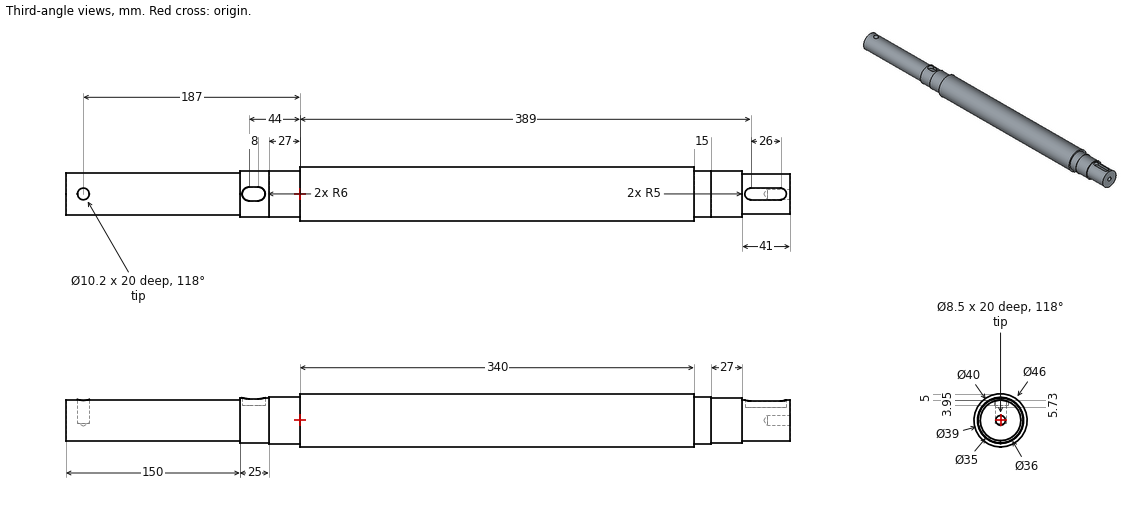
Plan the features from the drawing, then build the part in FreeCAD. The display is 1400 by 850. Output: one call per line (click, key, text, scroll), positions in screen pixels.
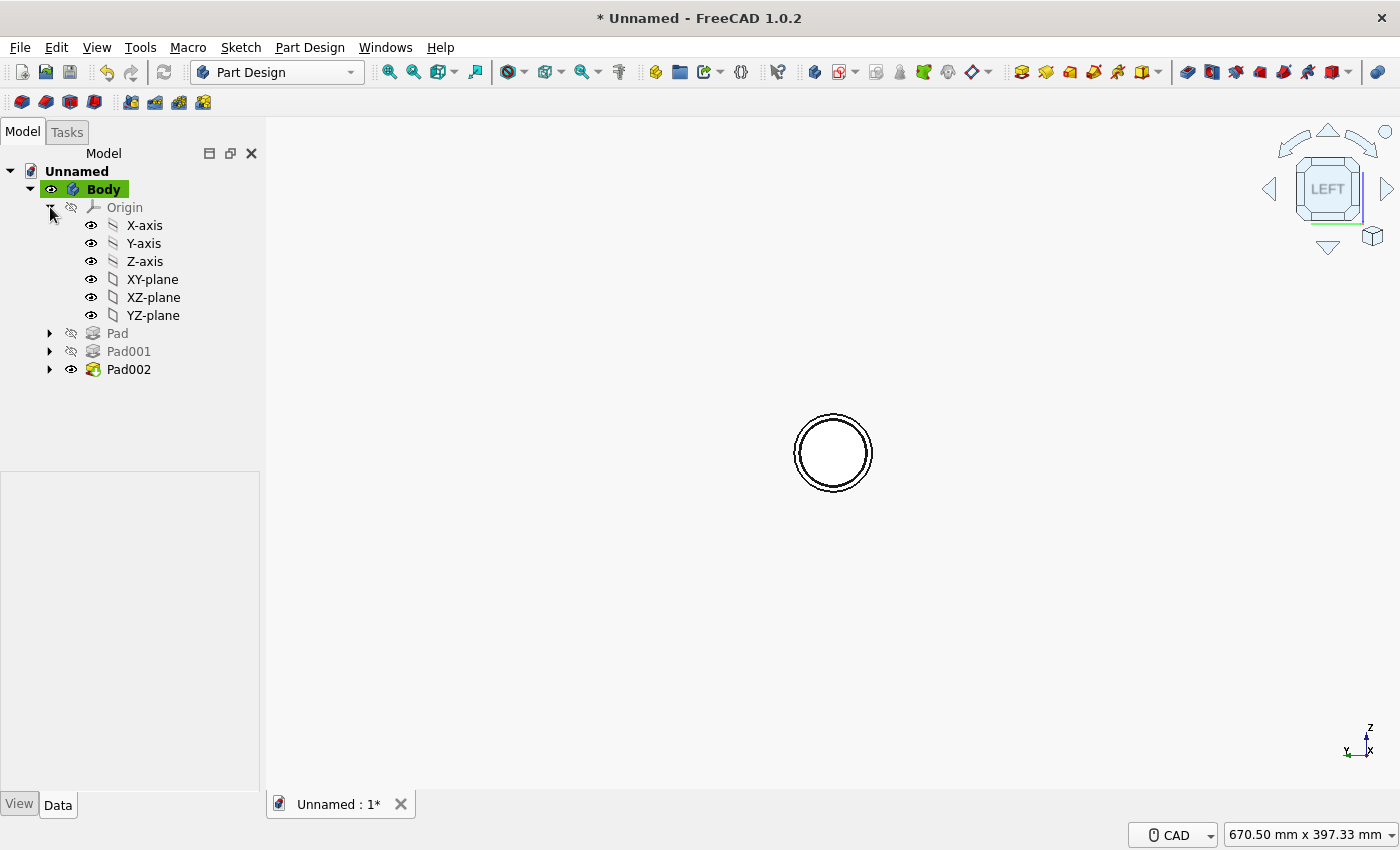
click(136, 315)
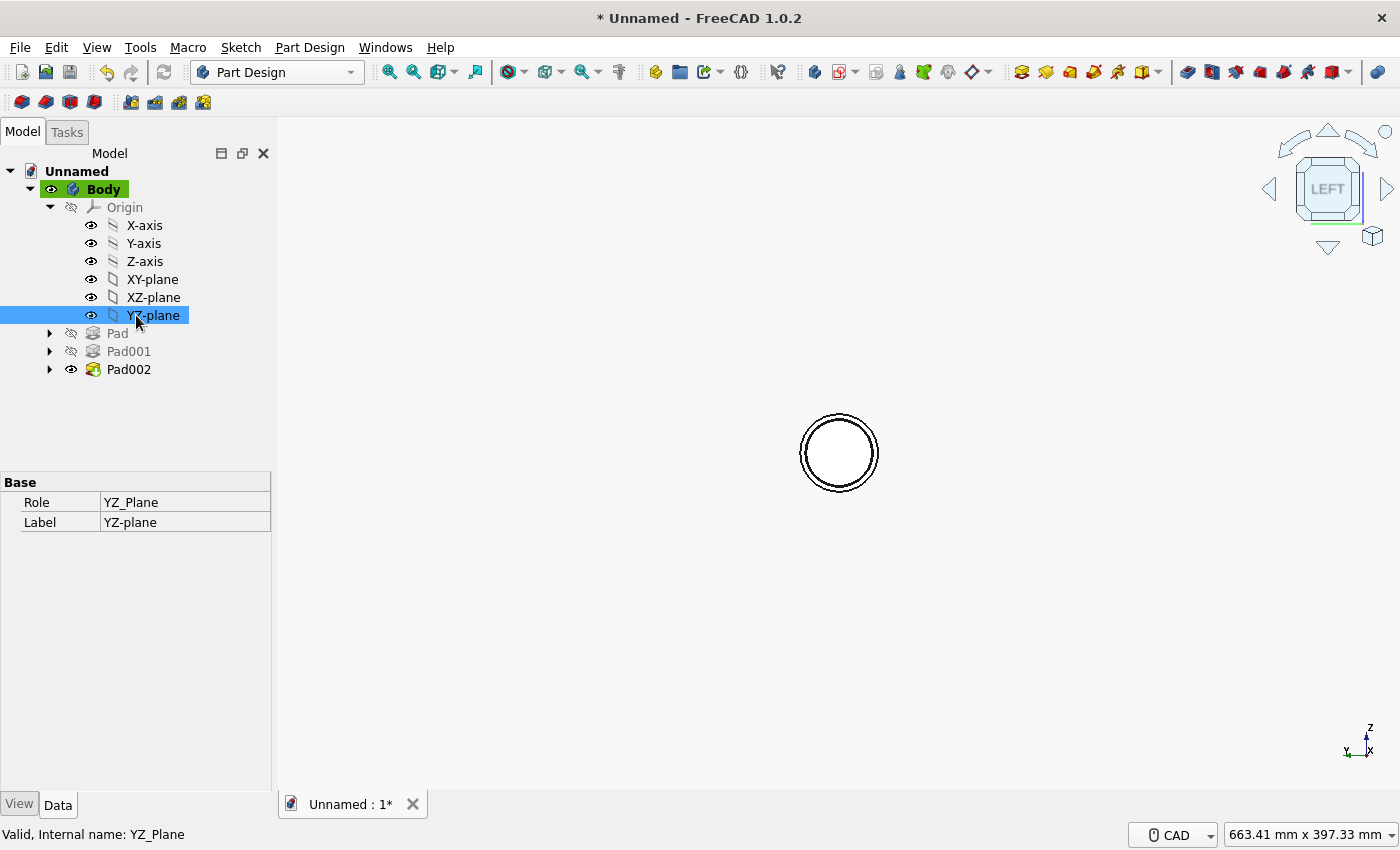
click(972, 72)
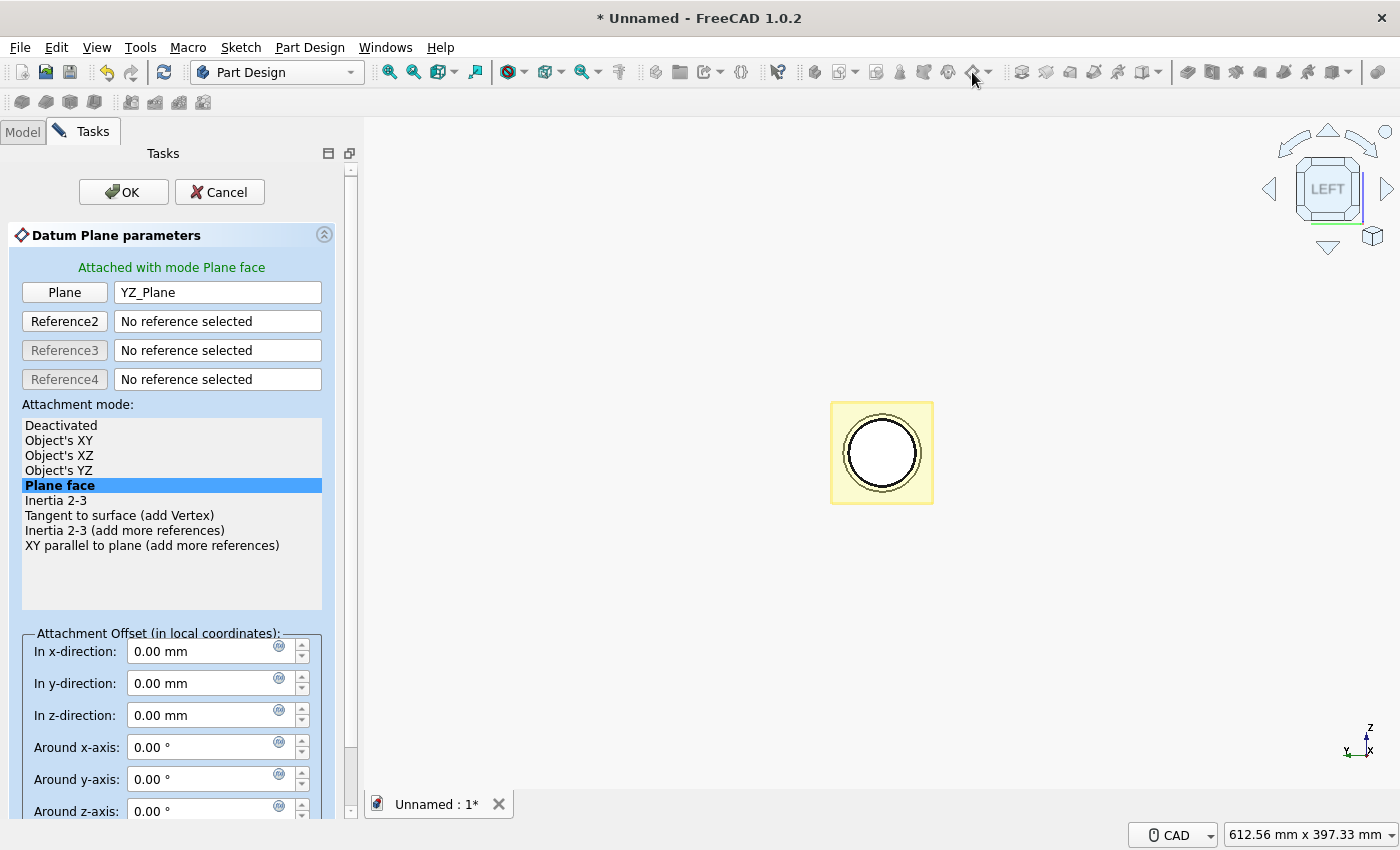
triple_click(210, 715)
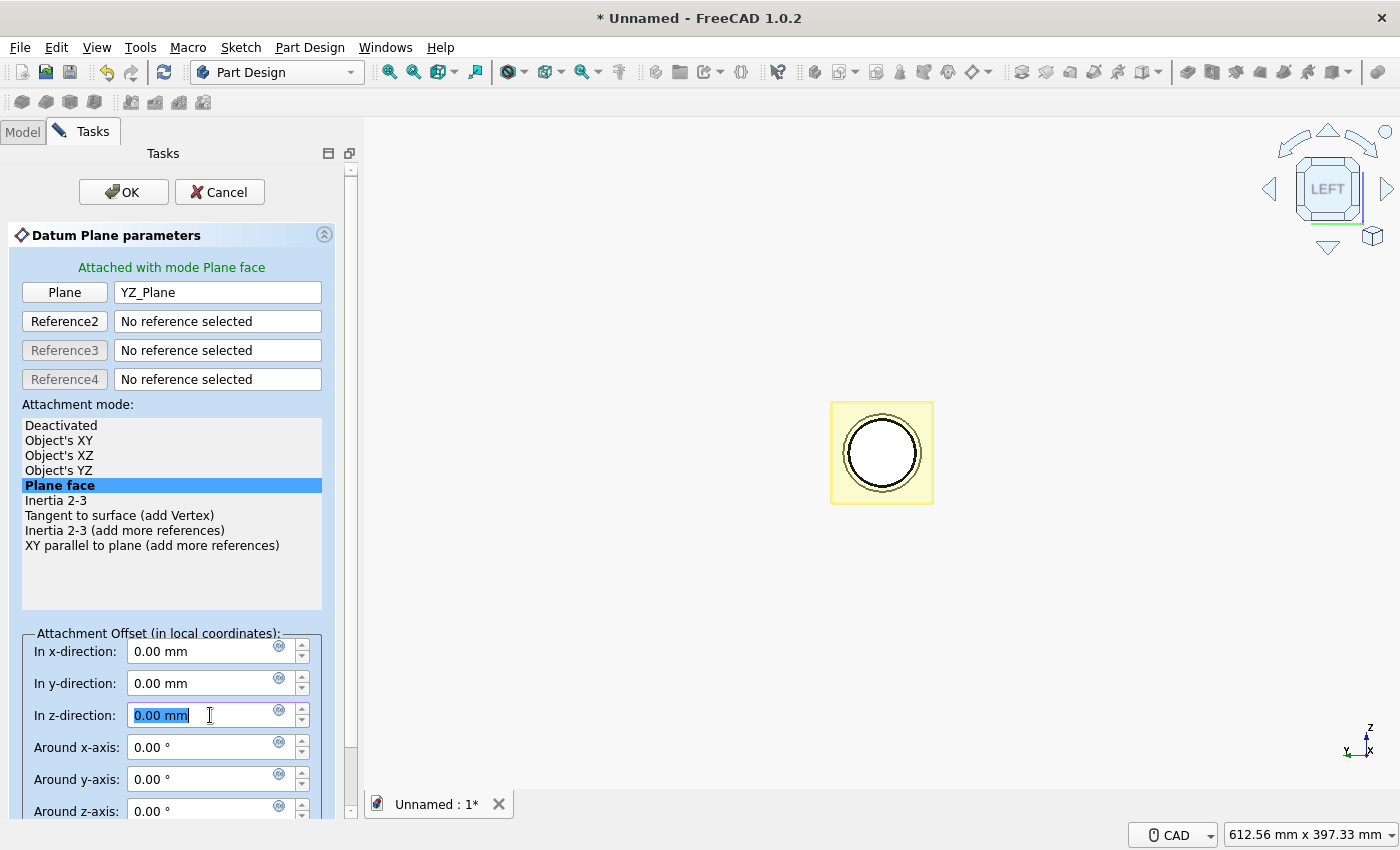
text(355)
key(Tab)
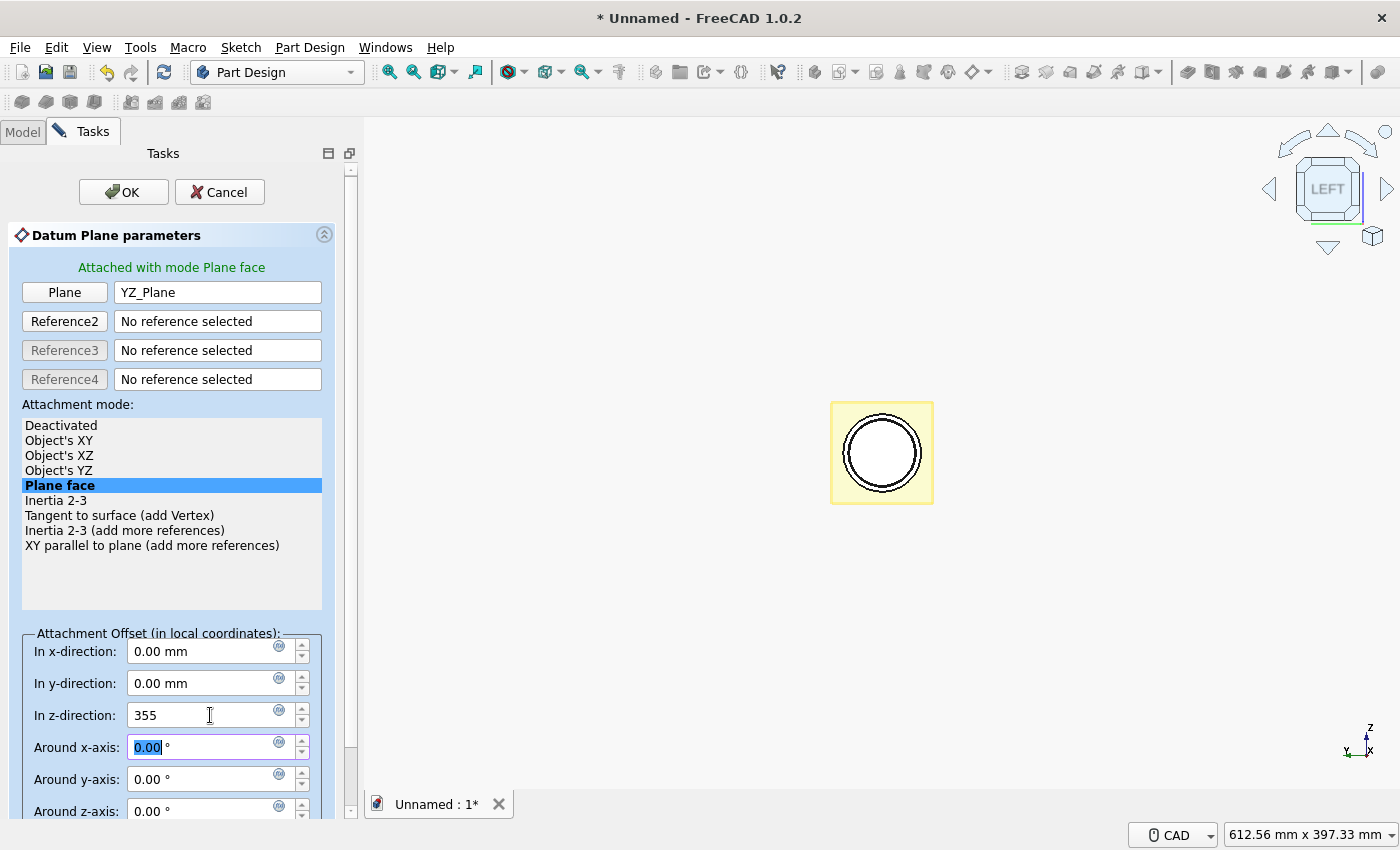
click(124, 192)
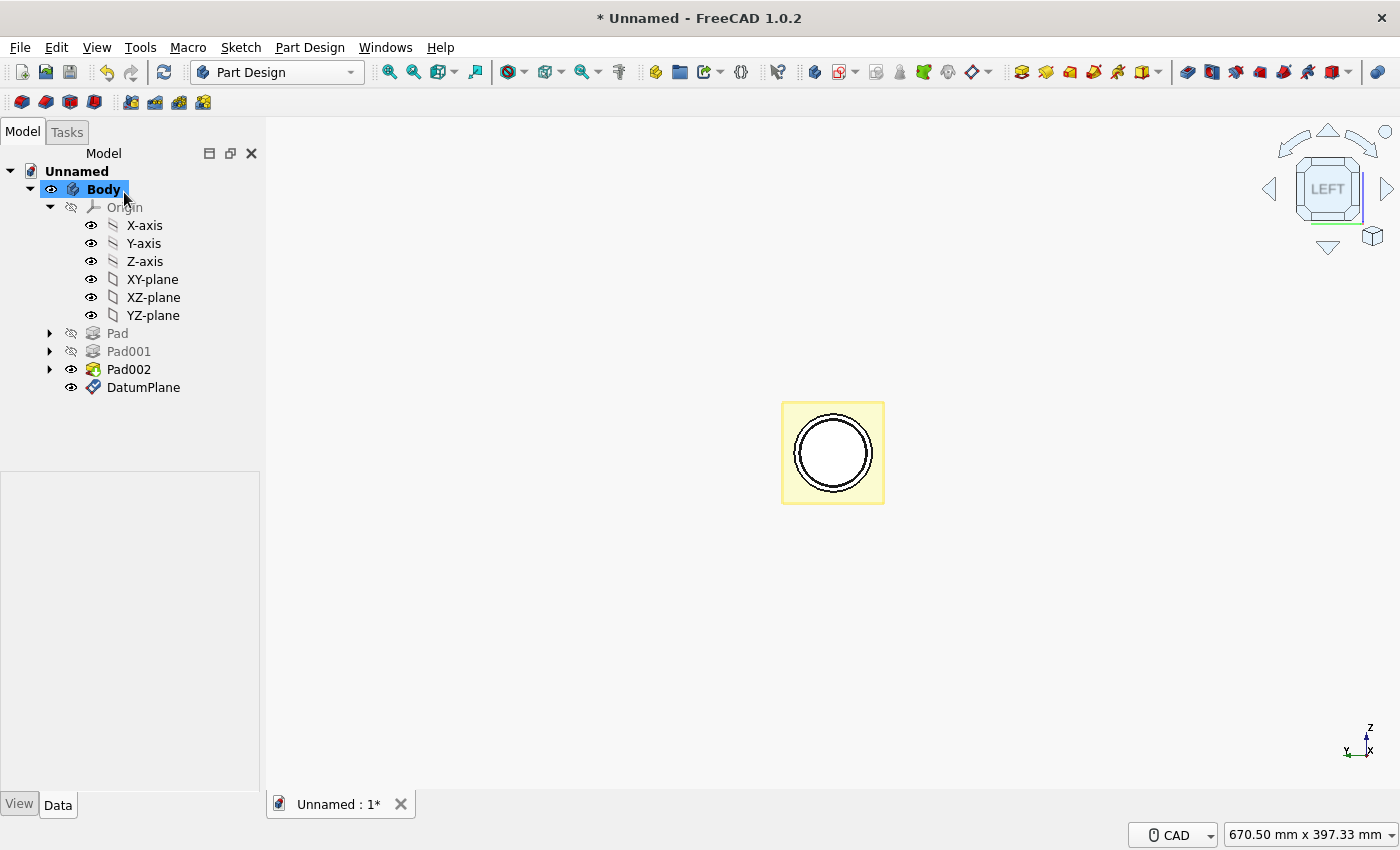
click(116, 387)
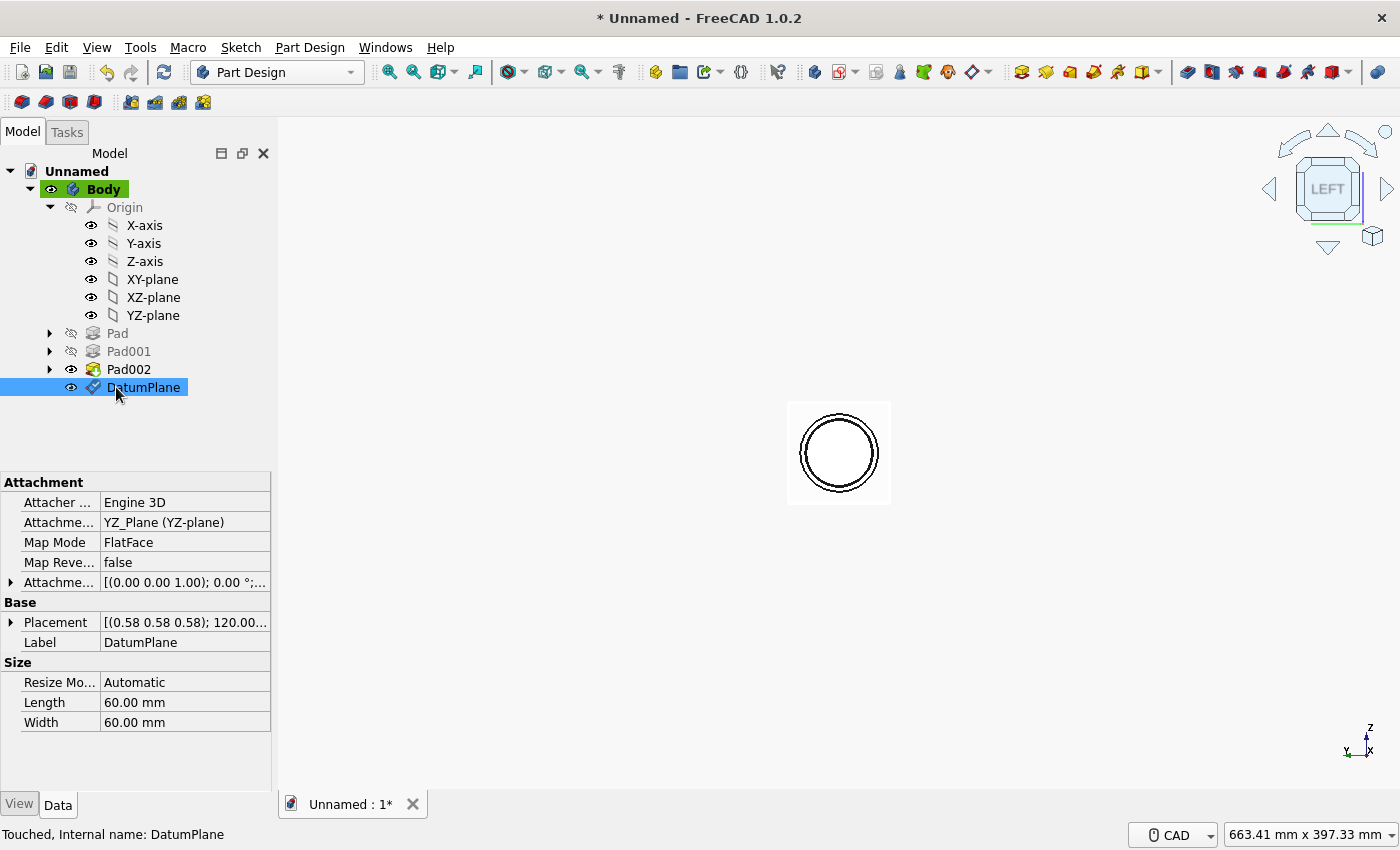
click(840, 72)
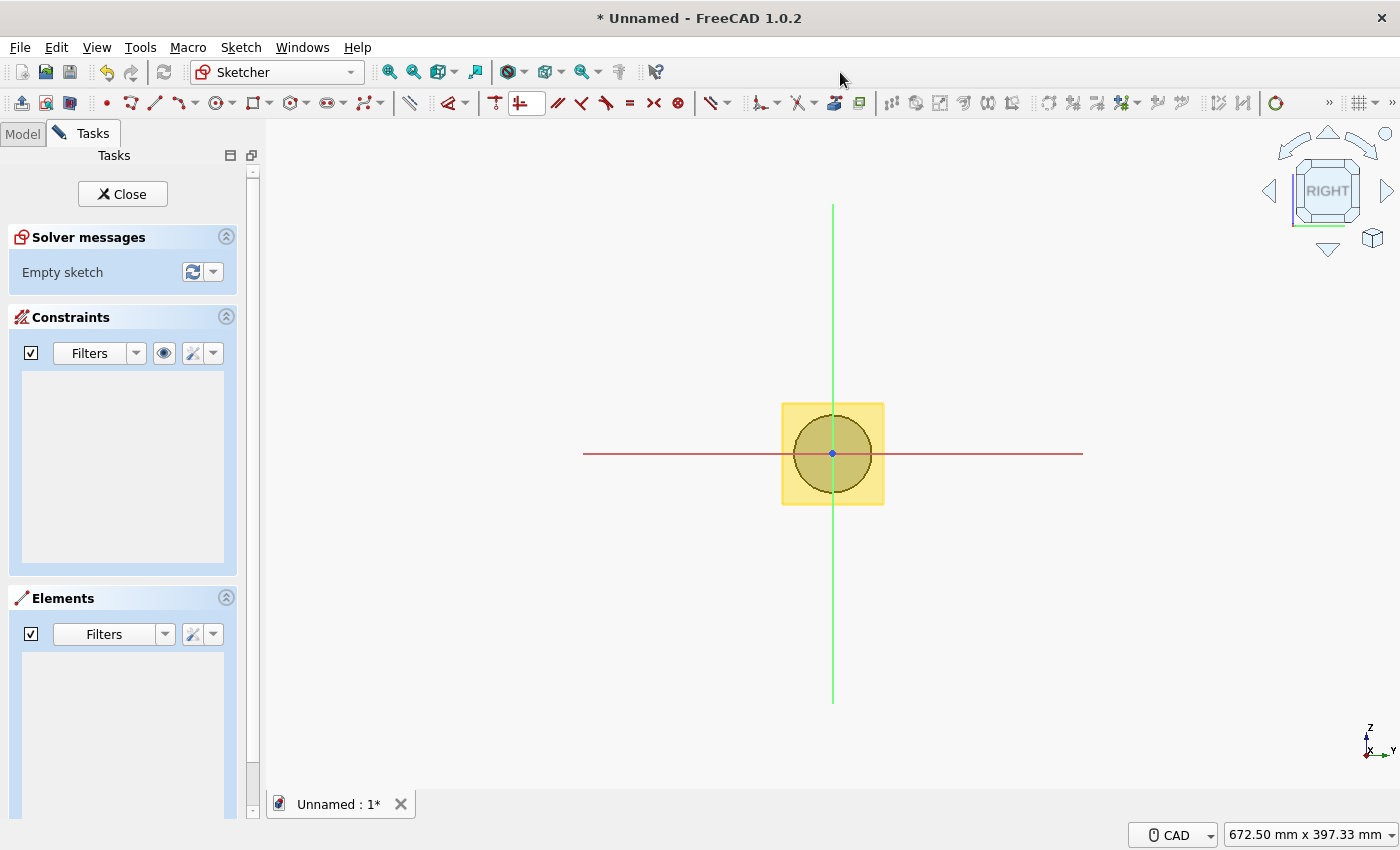
scroll(846, 454, up, 9)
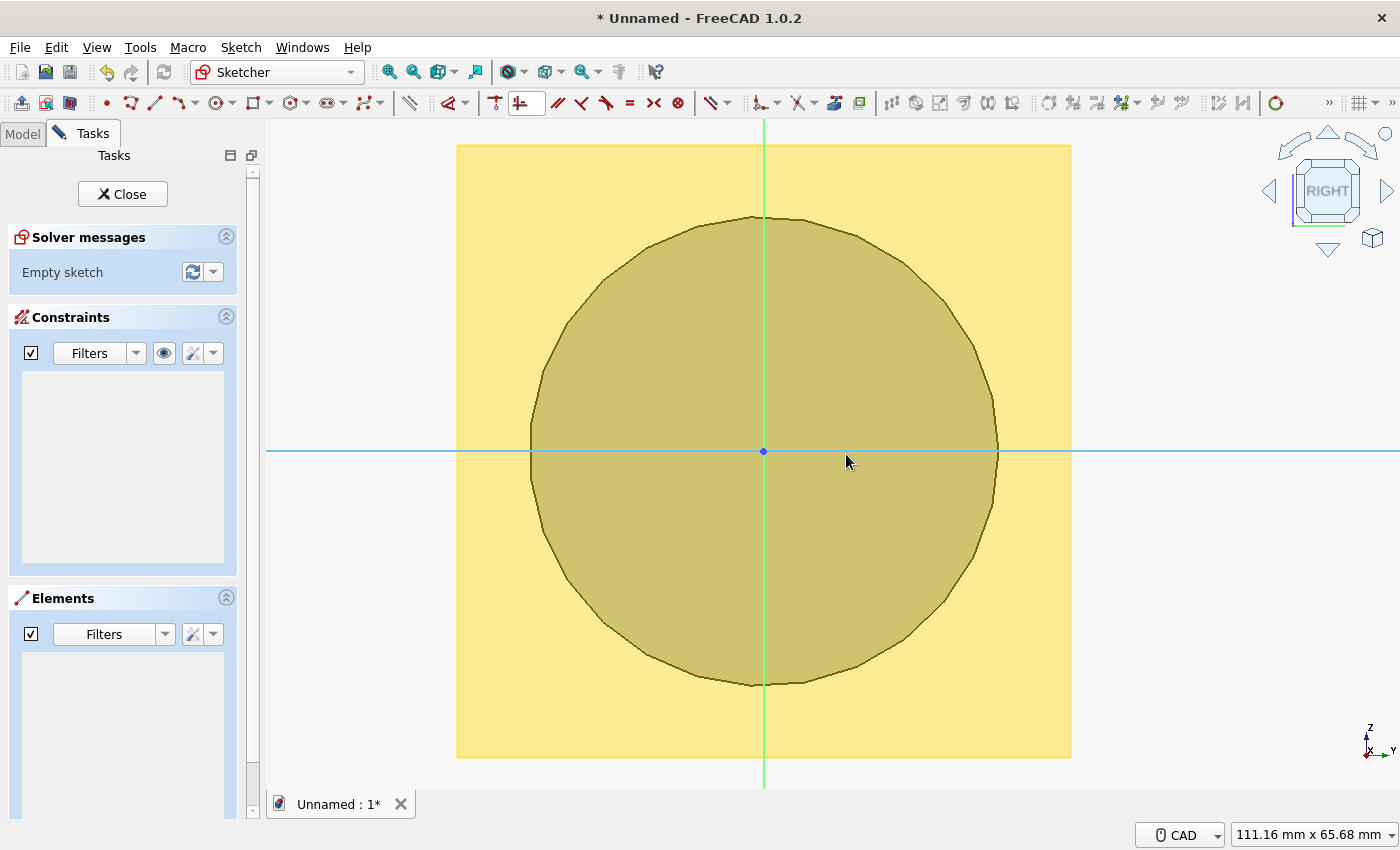
click(216, 104)